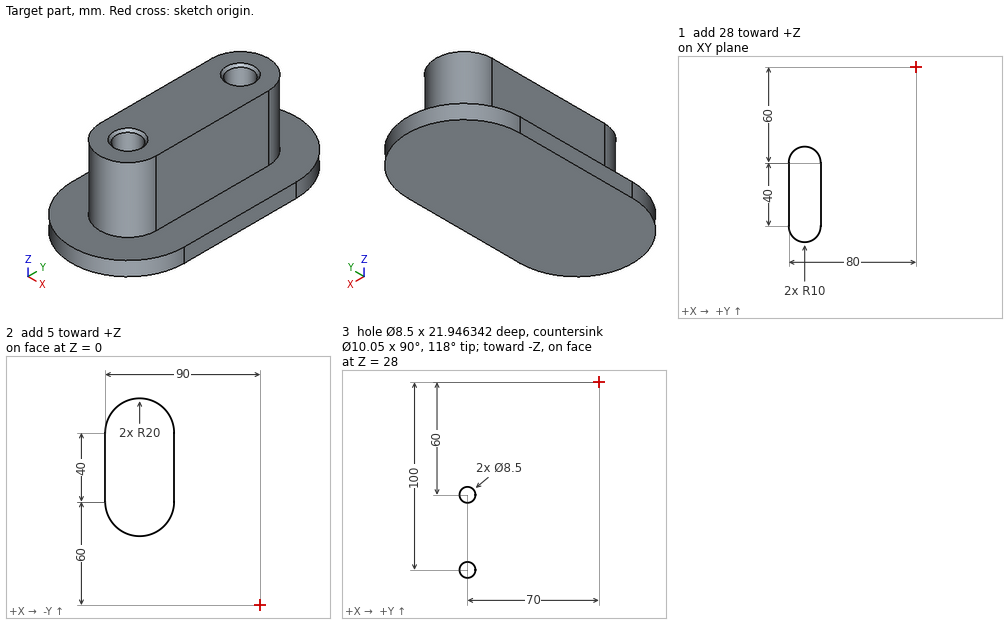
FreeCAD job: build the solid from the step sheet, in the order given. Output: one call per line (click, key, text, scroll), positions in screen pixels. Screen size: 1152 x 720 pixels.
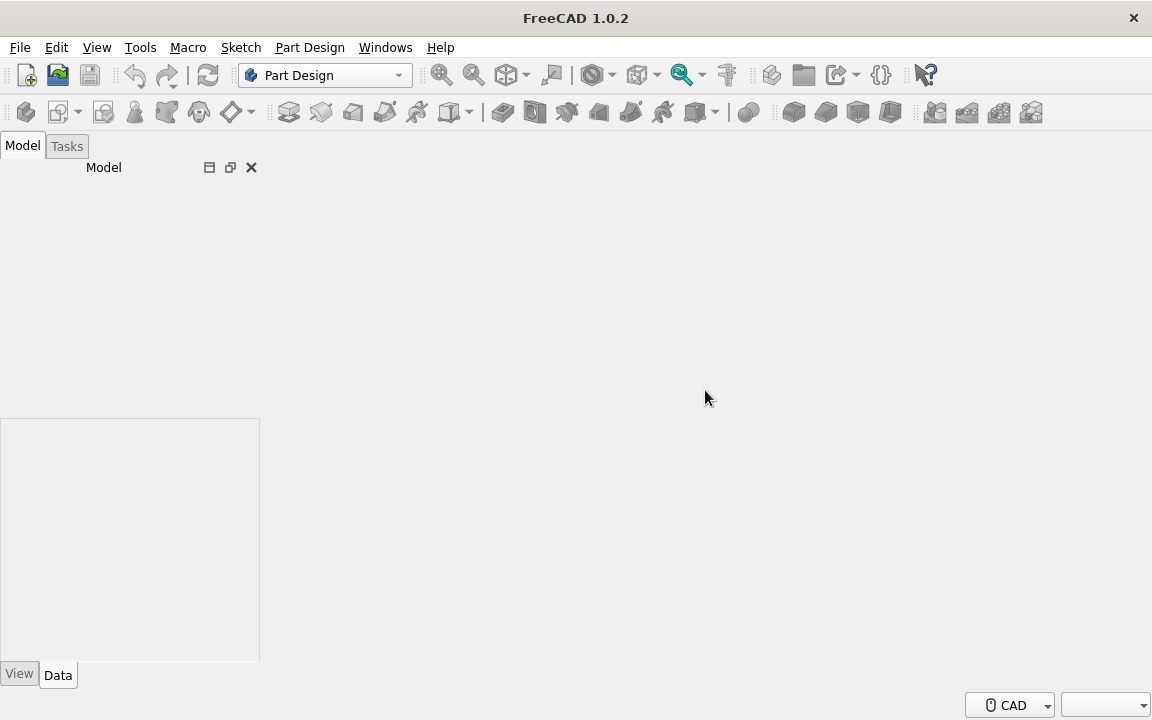
click(26, 76)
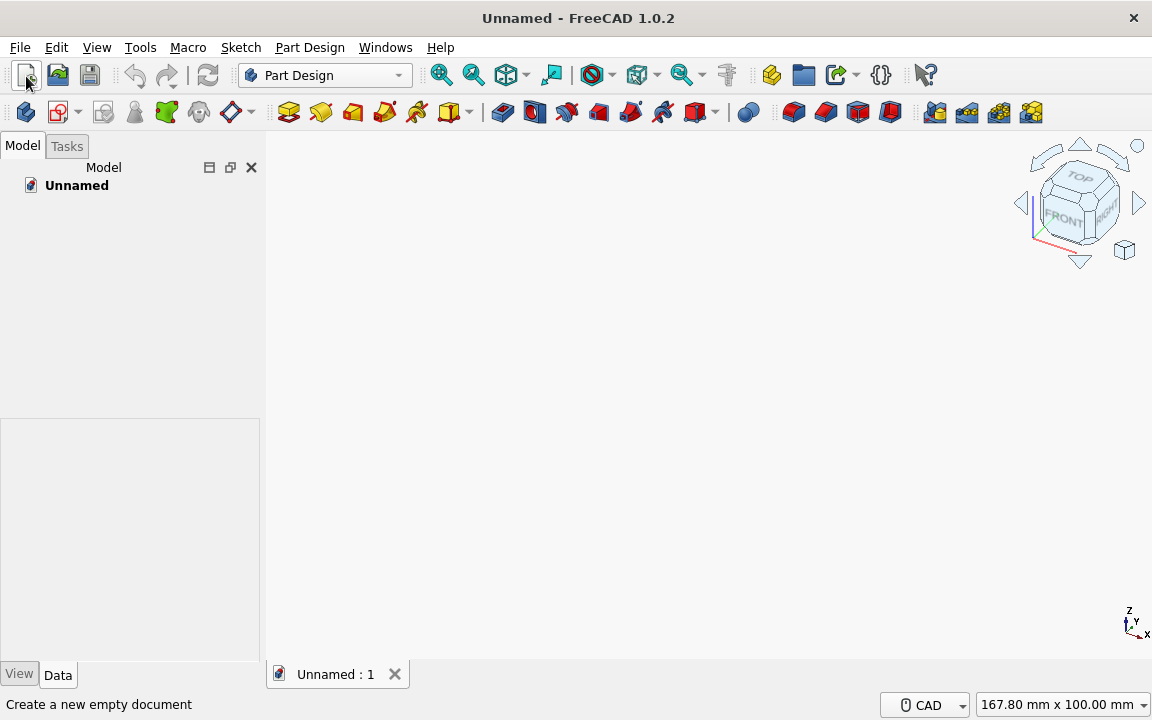
click(58, 112)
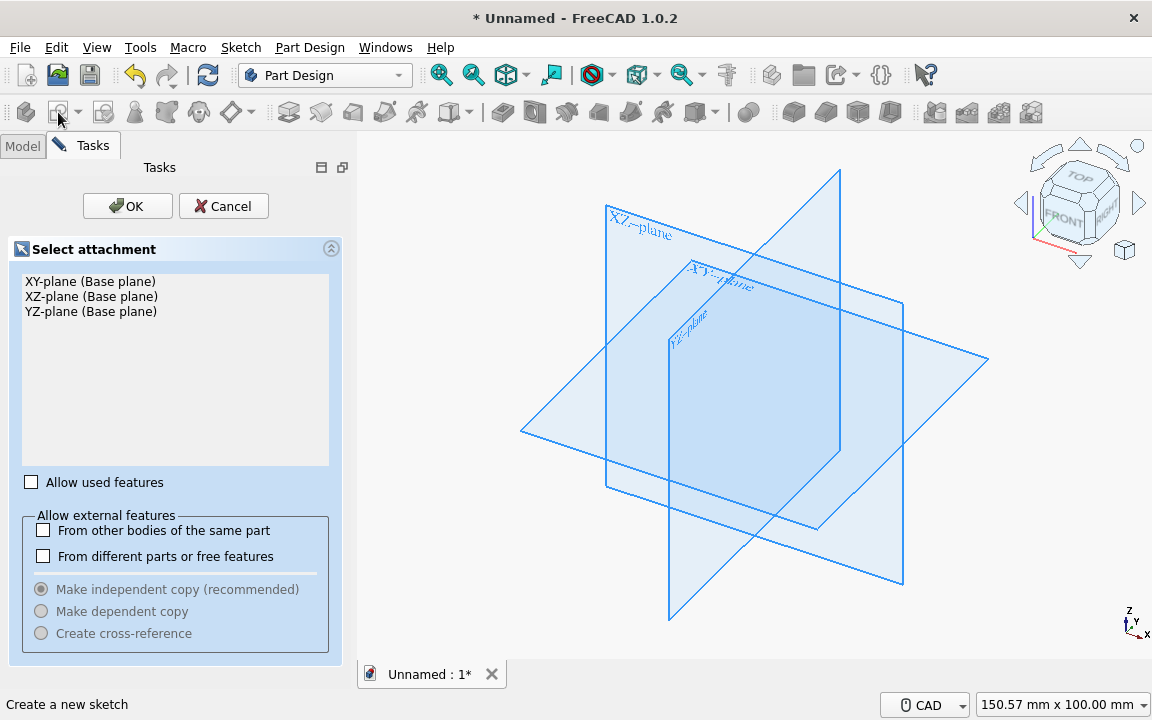
click(82, 282)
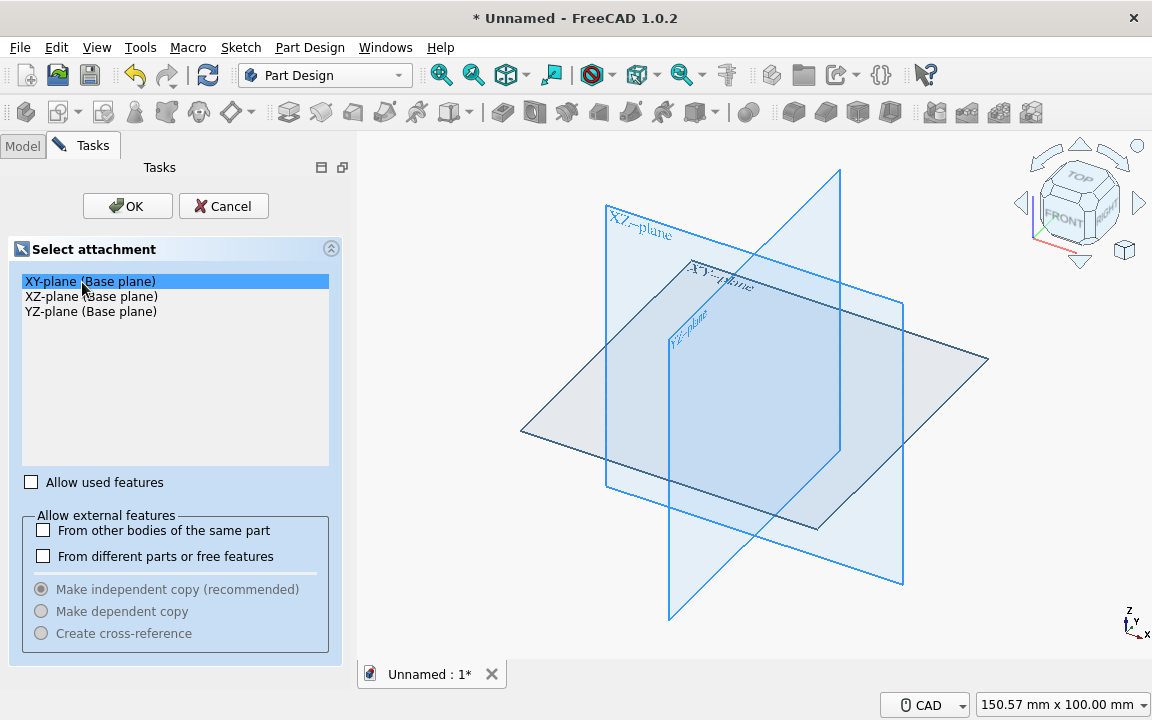
click(128, 206)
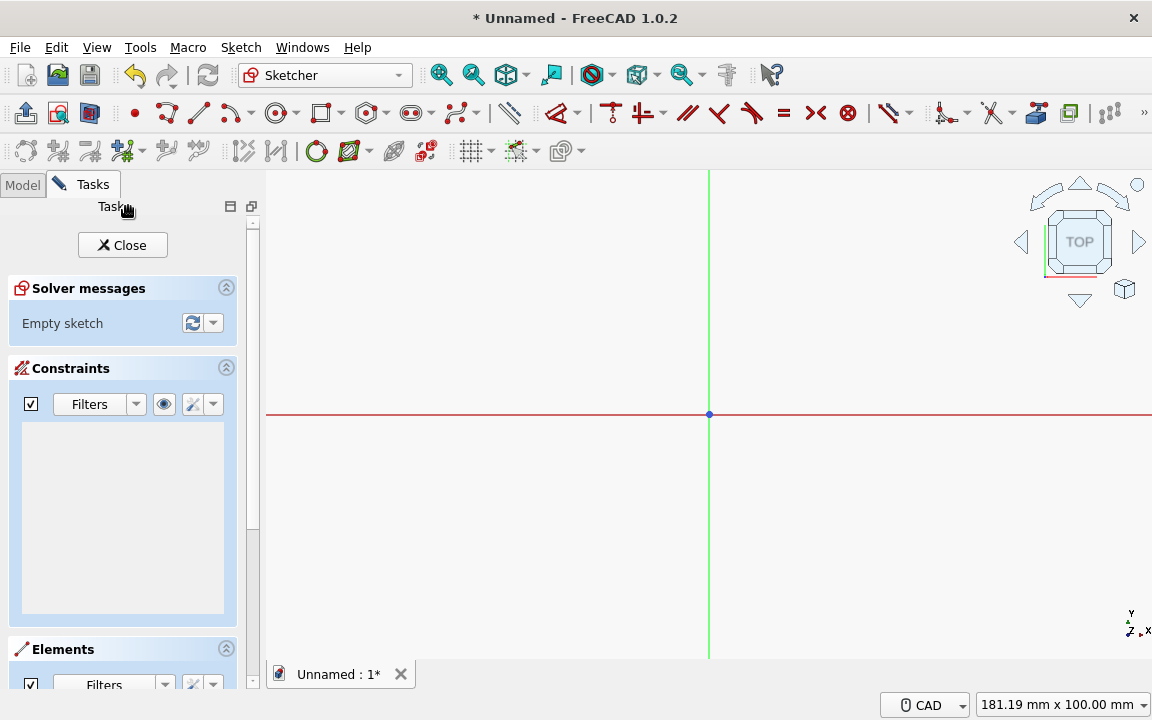
scroll(744, 198, down, 4)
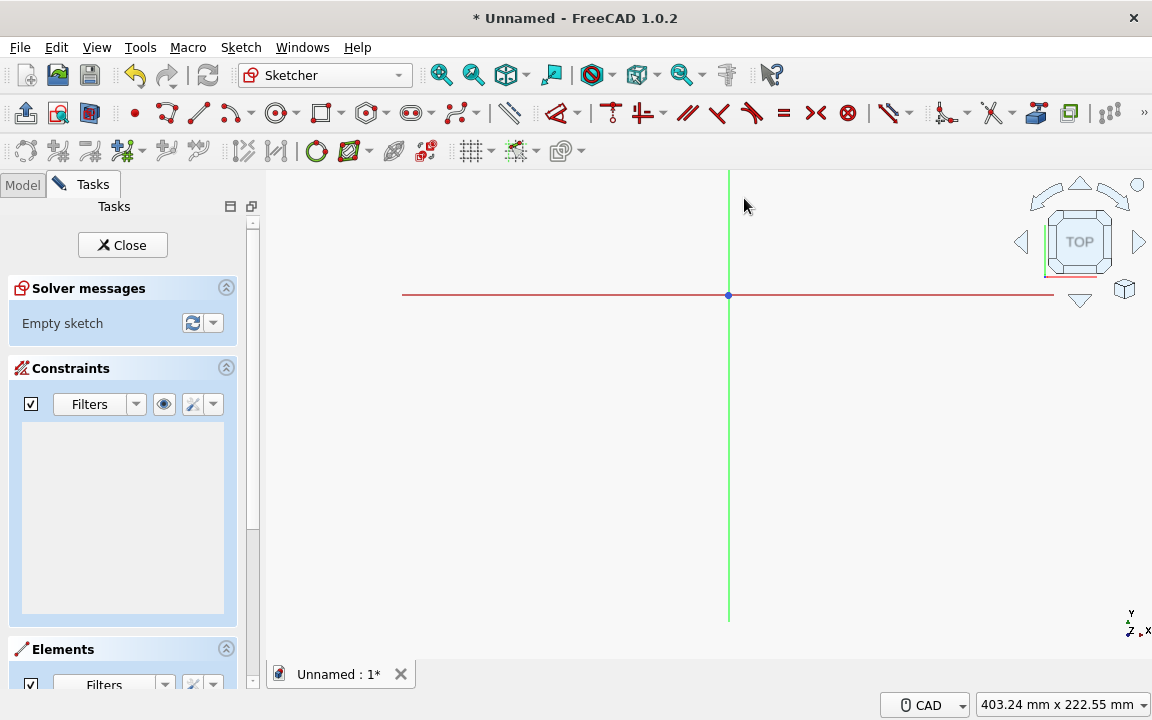
click(412, 114)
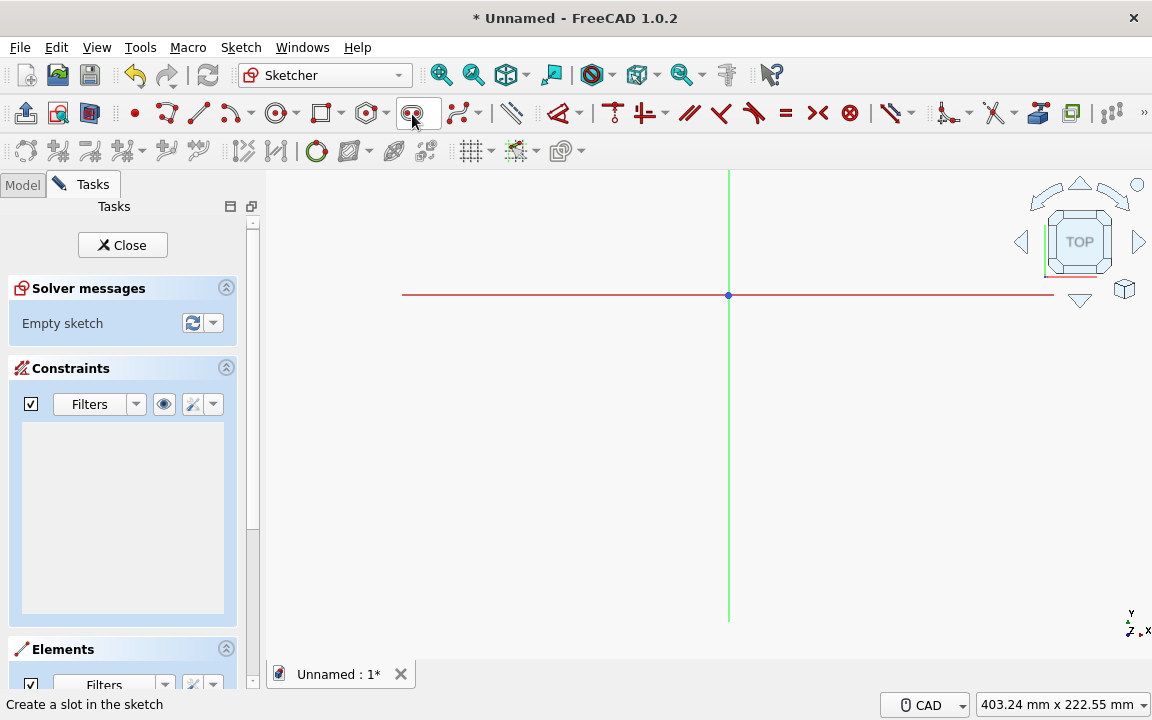
click(575, 515)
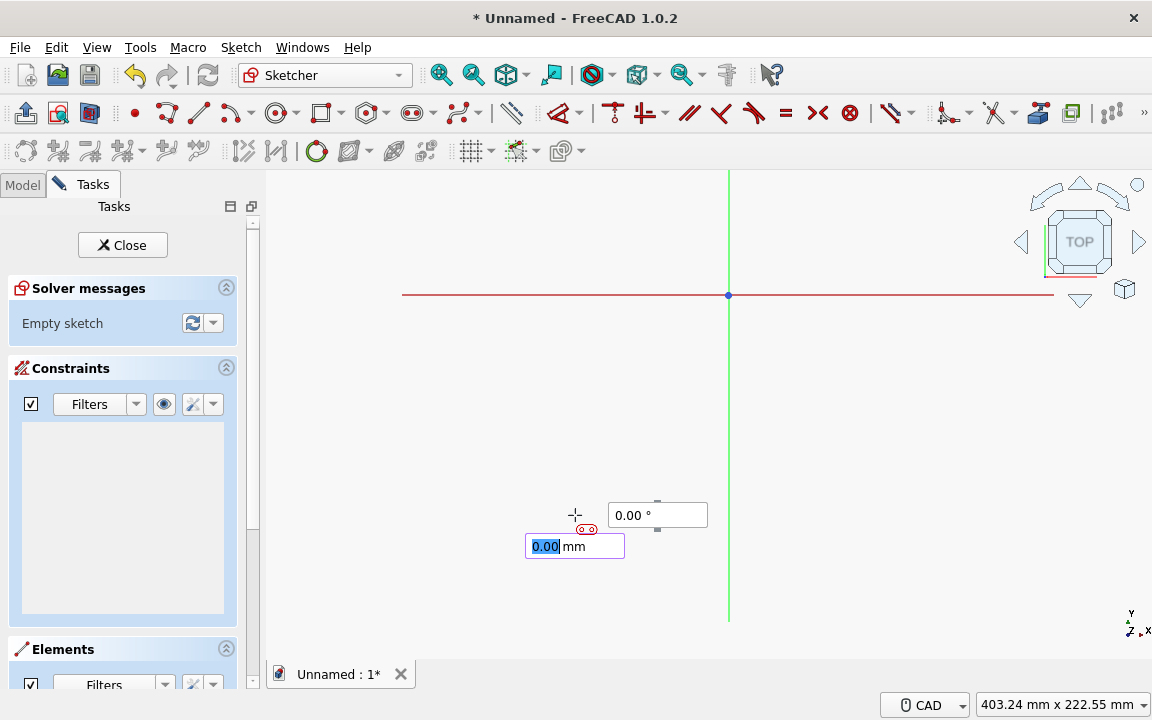
click(575, 427)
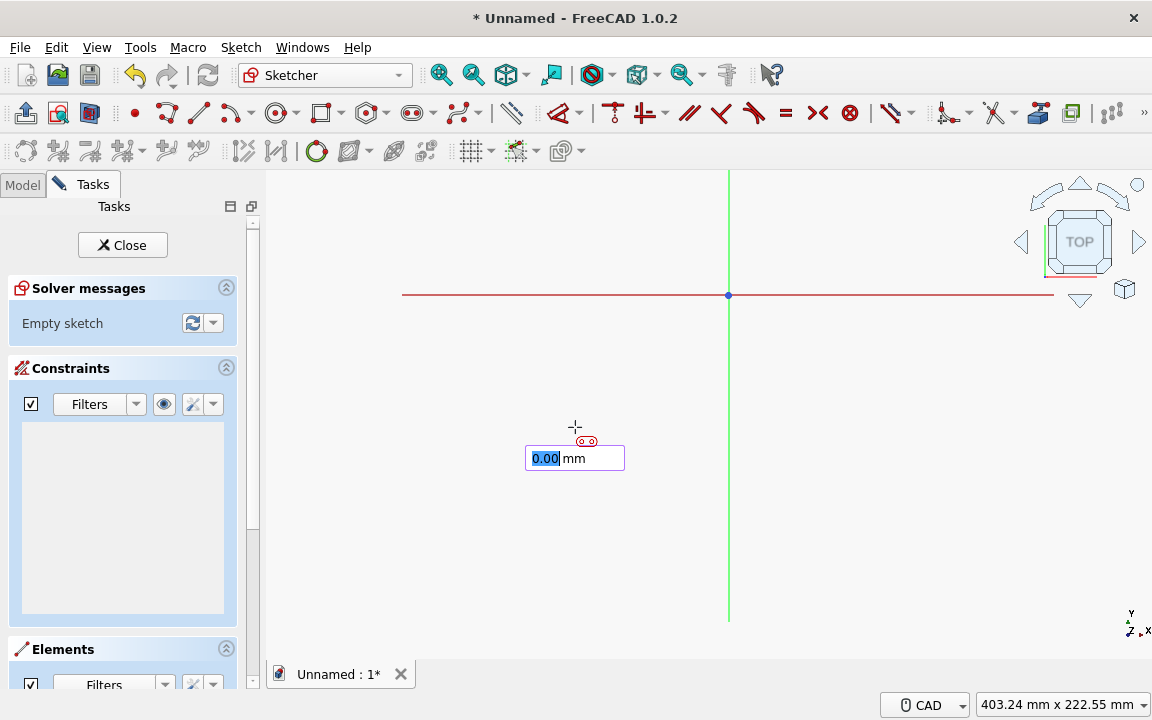
click(597, 471)
key(Escape)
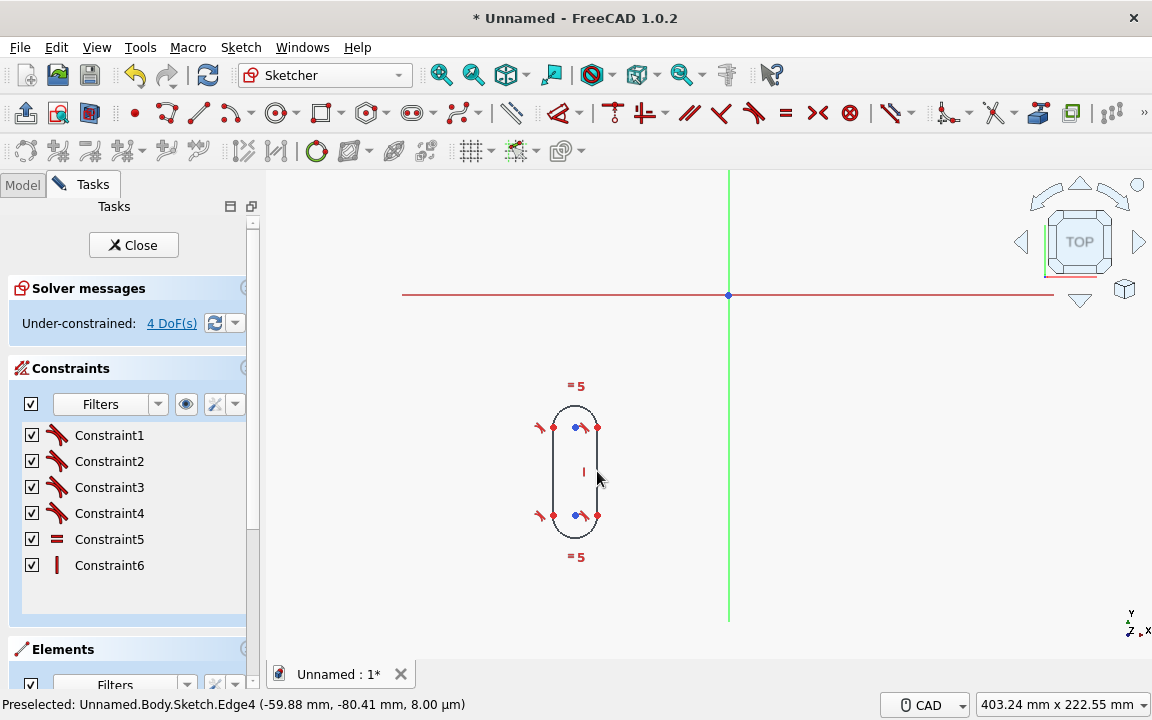
click(558, 114)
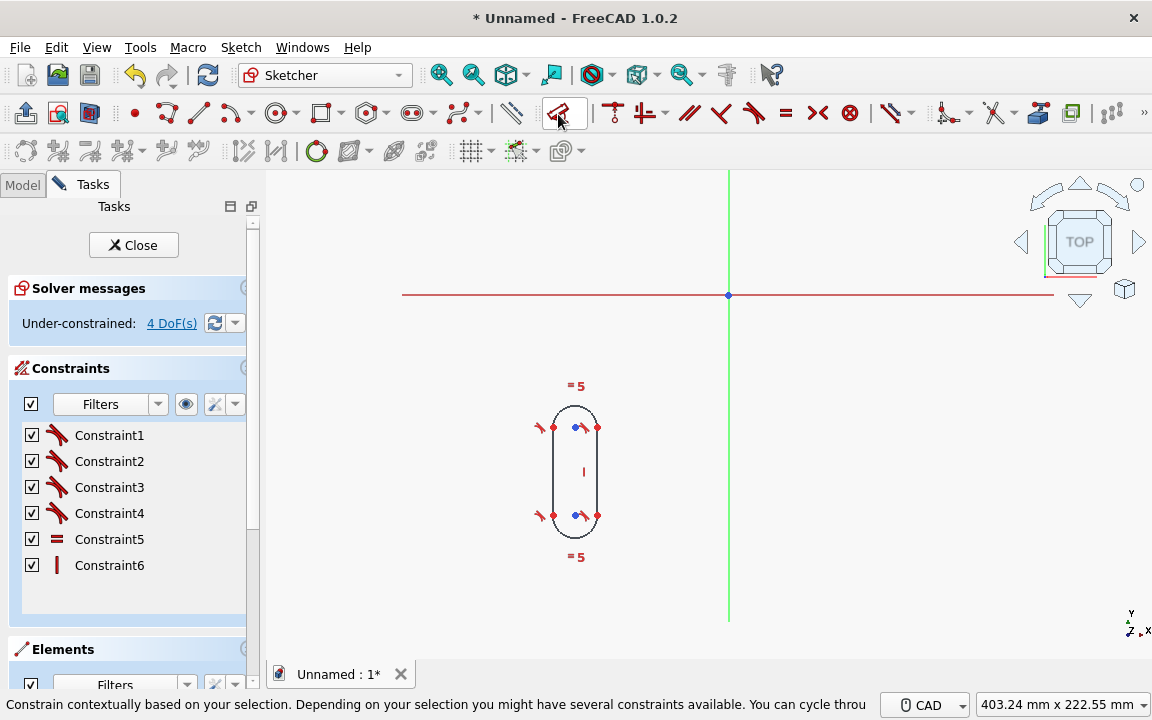
scroll(562, 534, up, 3)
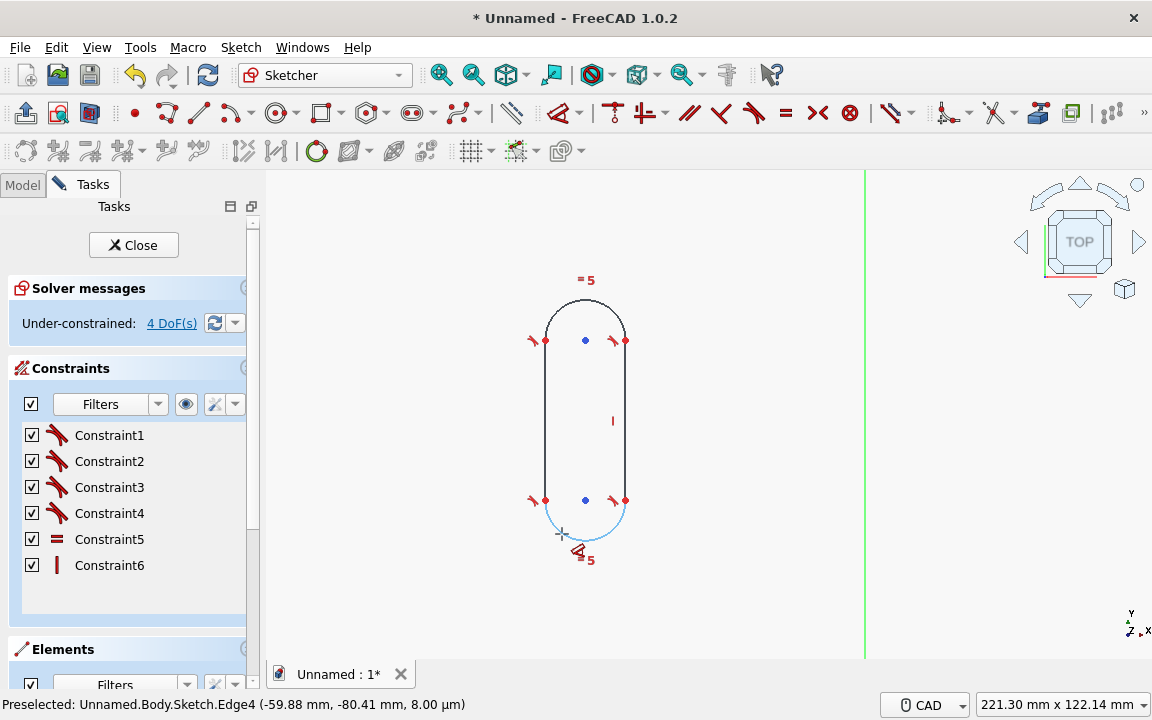
click(562, 533)
click(543, 559)